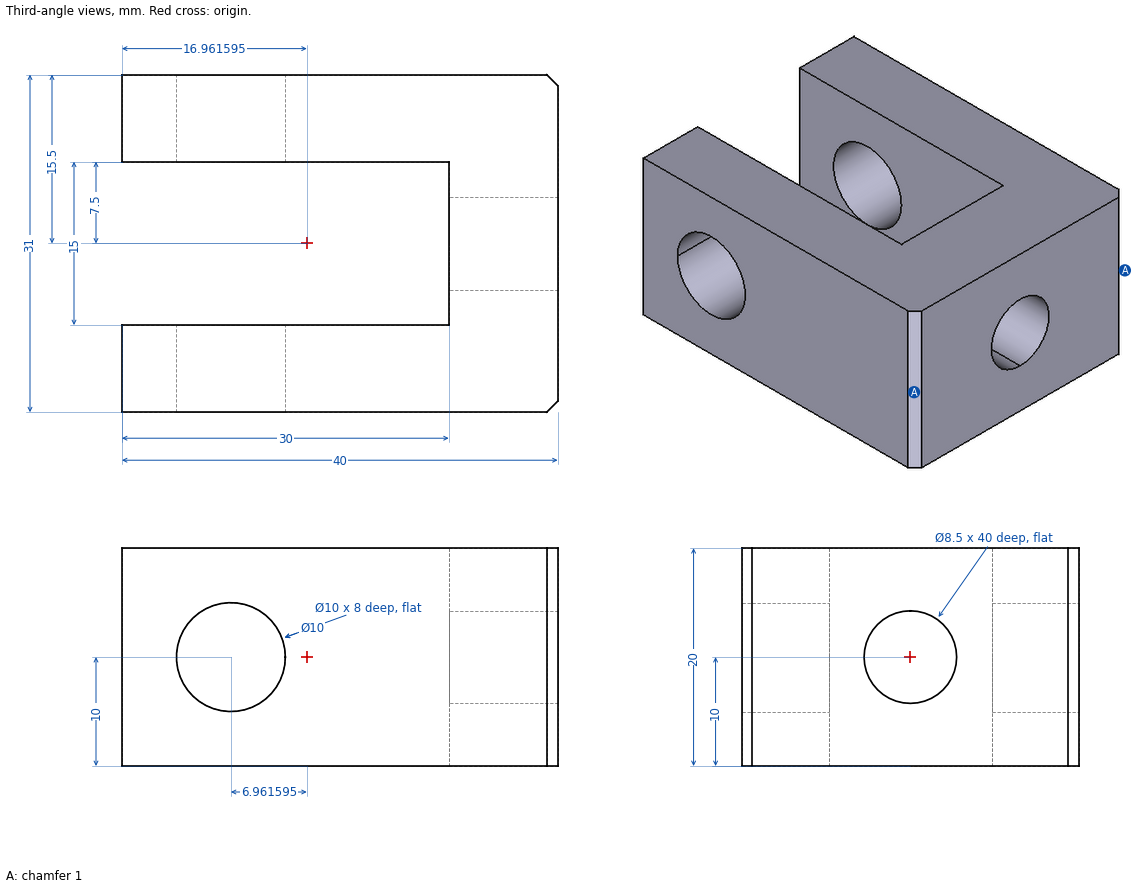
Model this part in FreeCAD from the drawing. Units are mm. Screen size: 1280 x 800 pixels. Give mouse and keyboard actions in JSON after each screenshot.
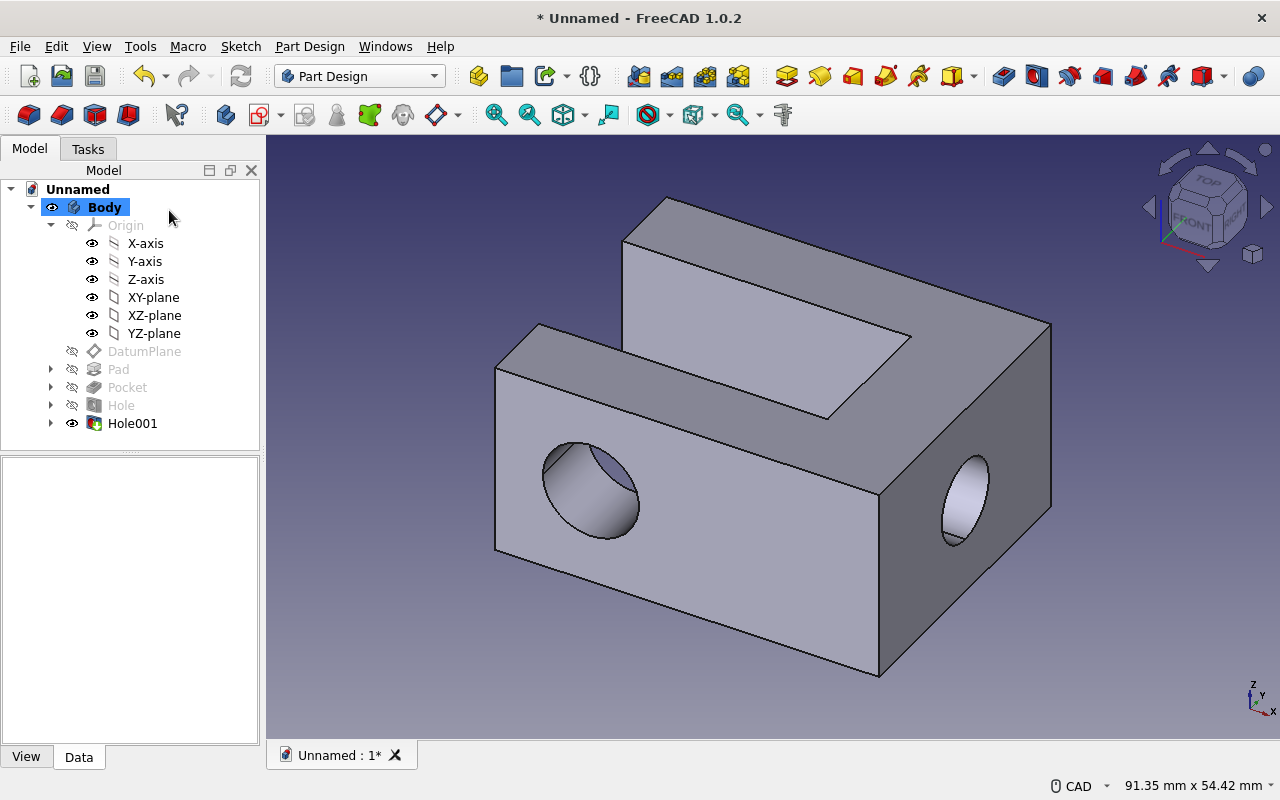
{"action": "left_click", "coordinate": [725, 365]}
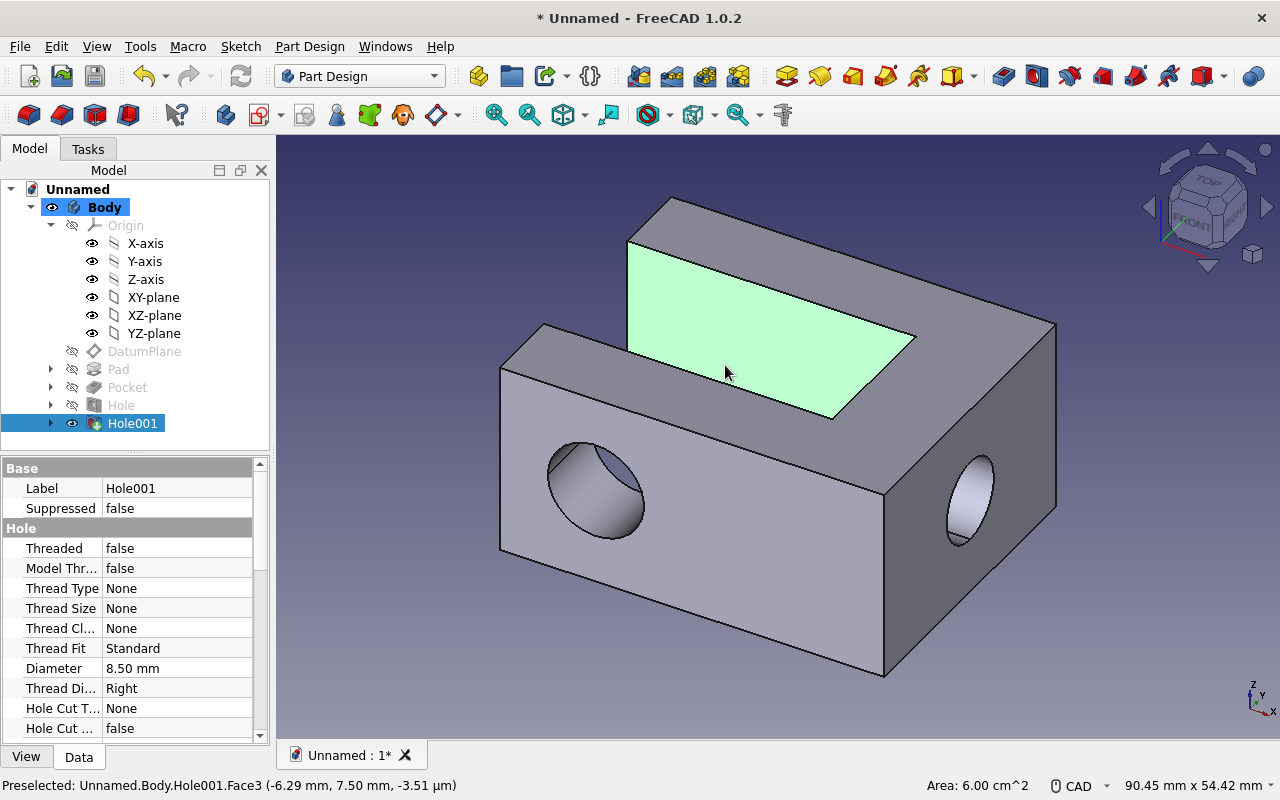
{"action": "left_click", "coordinate": [258, 116]}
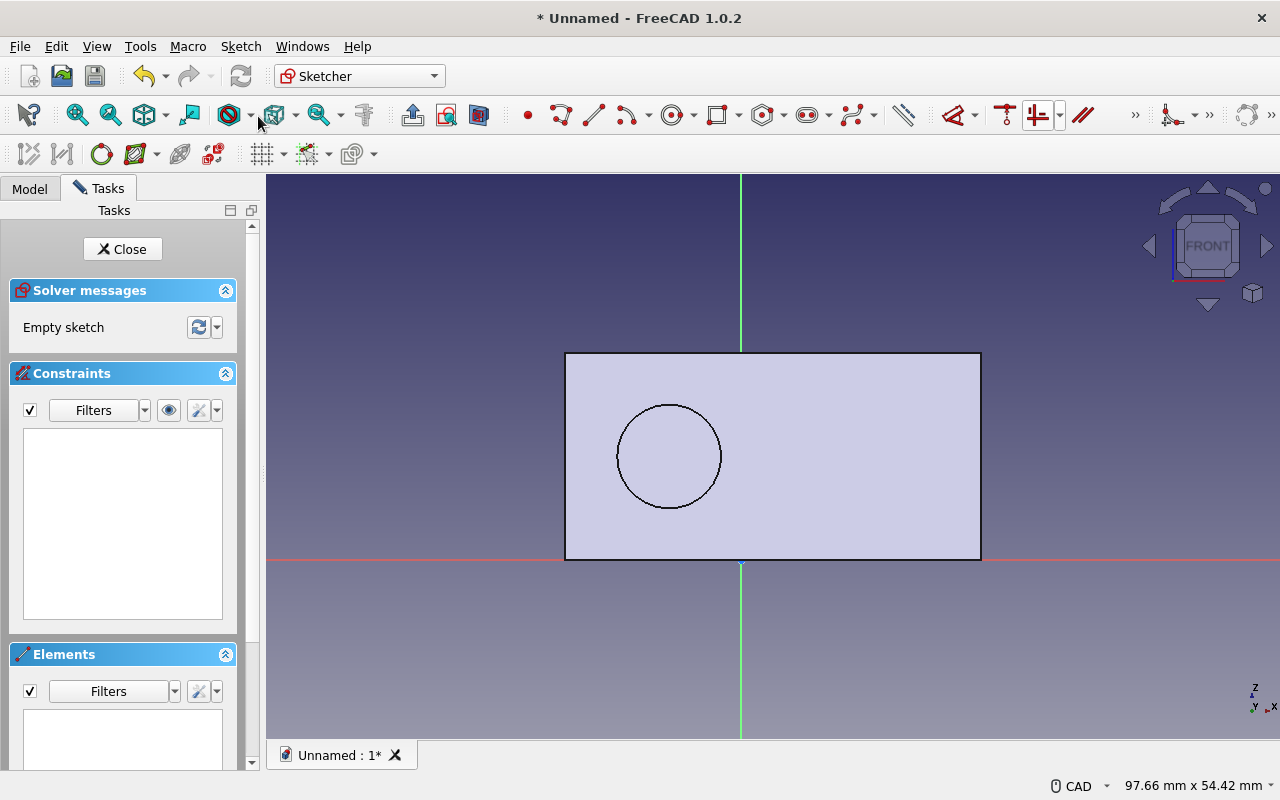
{"action": "scroll", "coordinate": [659, 504], "scroll_direction": "up", "scroll_amount": 4}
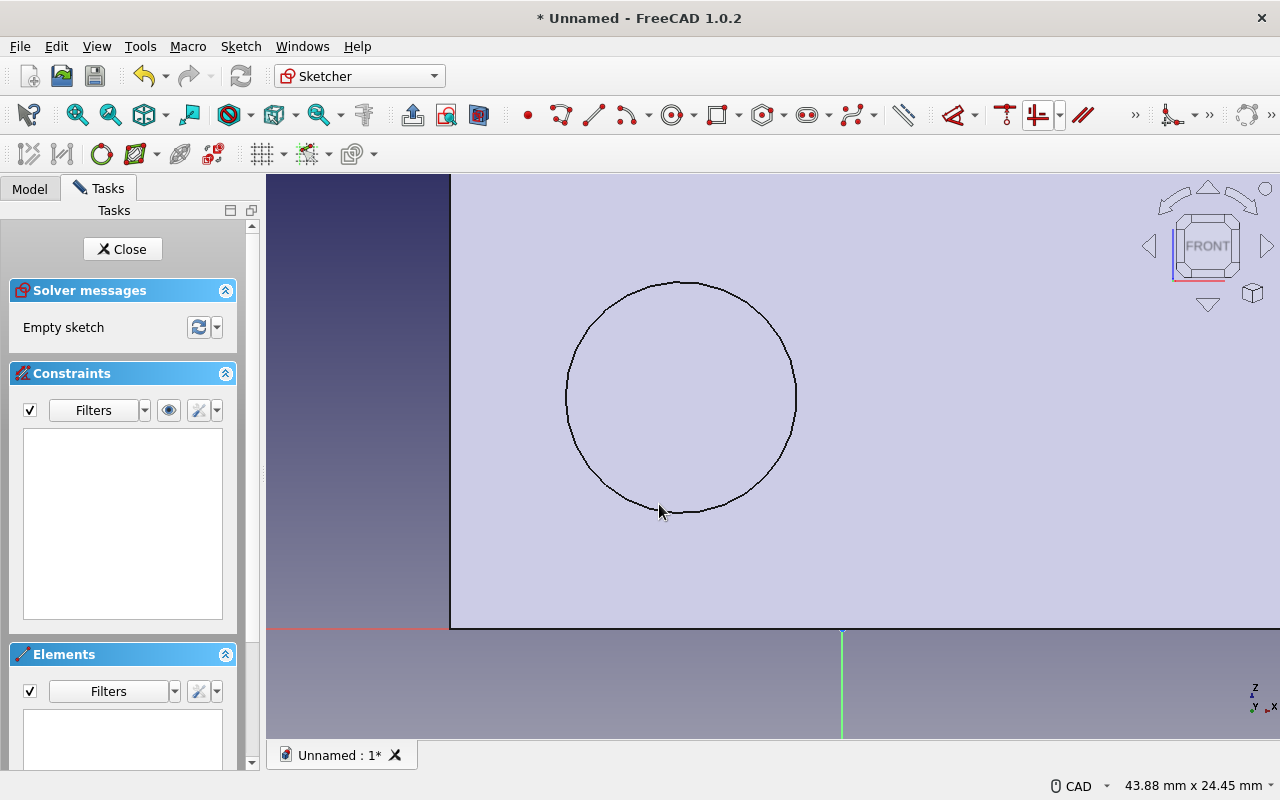
{"action": "key", "text": "g c"}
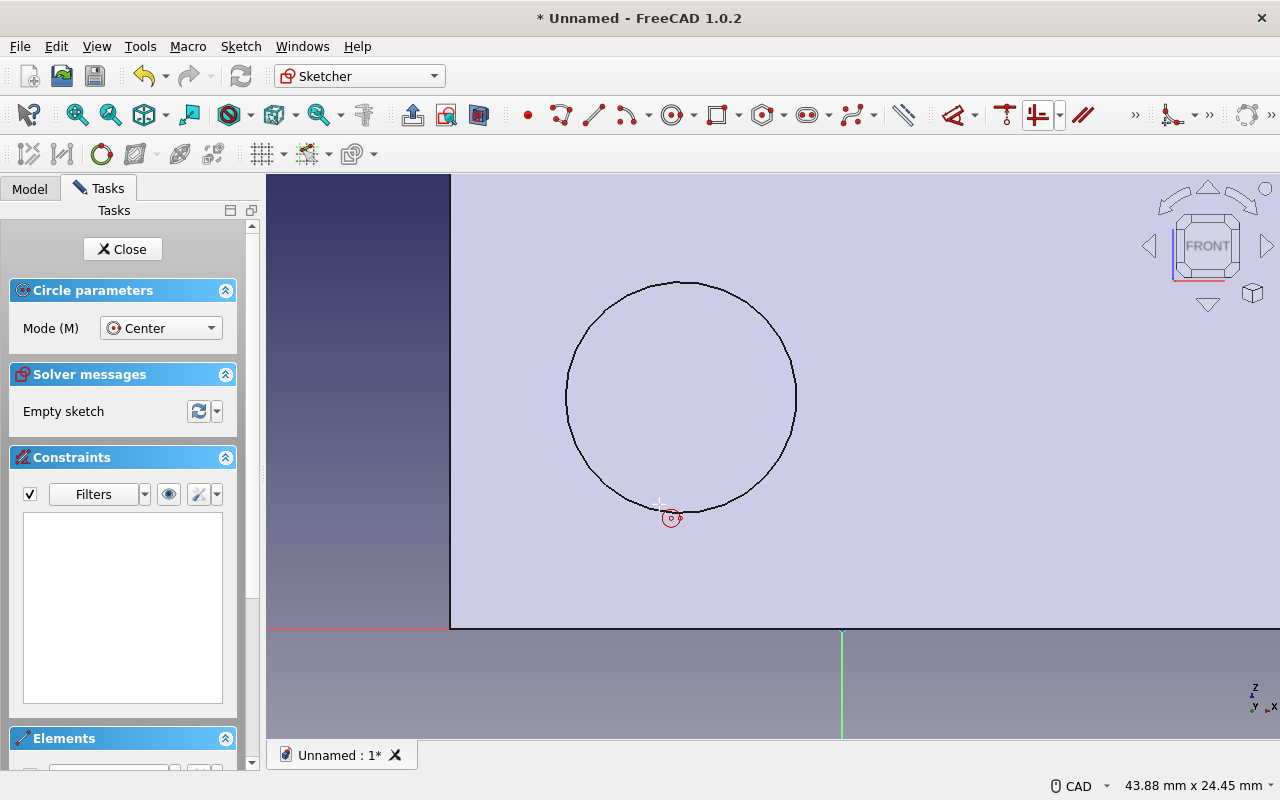
{"action": "left_click", "coordinate": [681, 398]}
{"action": "left_click", "coordinate": [763, 316]}
{"action": "key", "text": "Escape"}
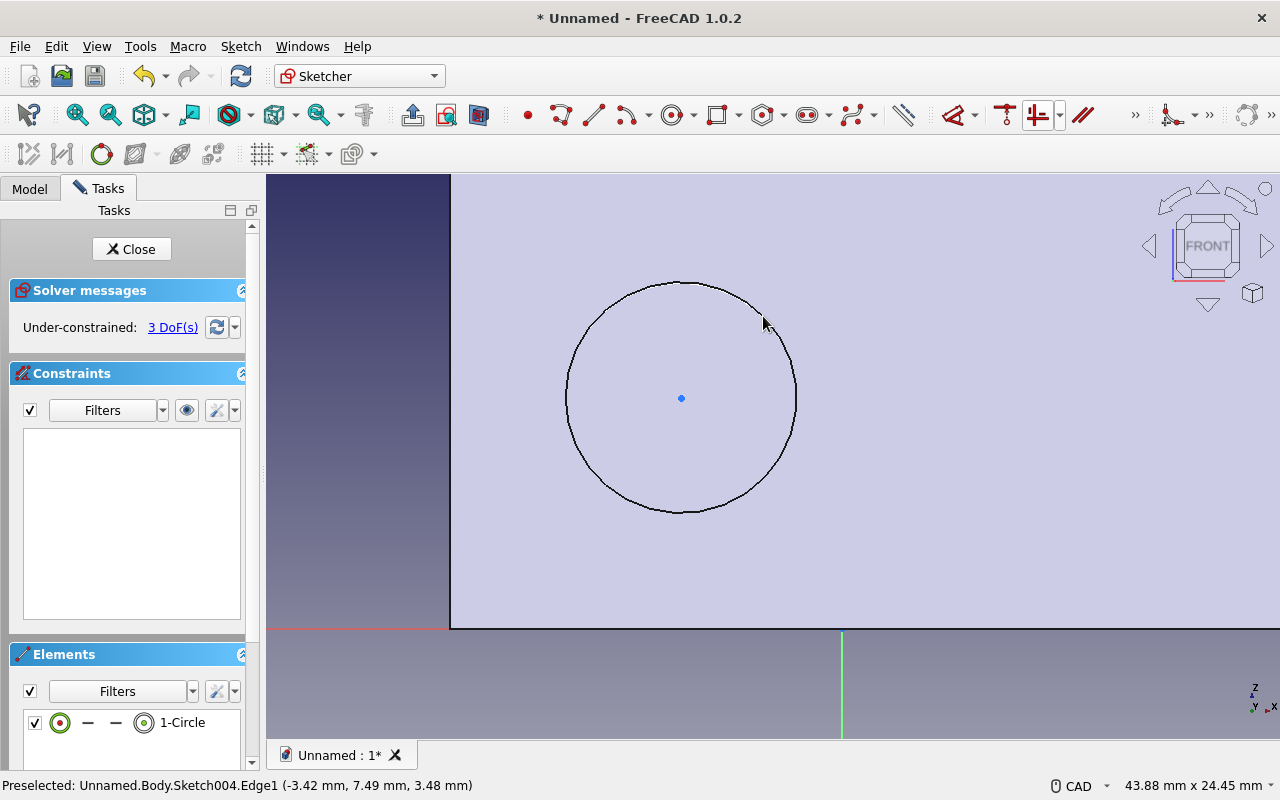
{"action": "left_click", "coordinate": [952, 116]}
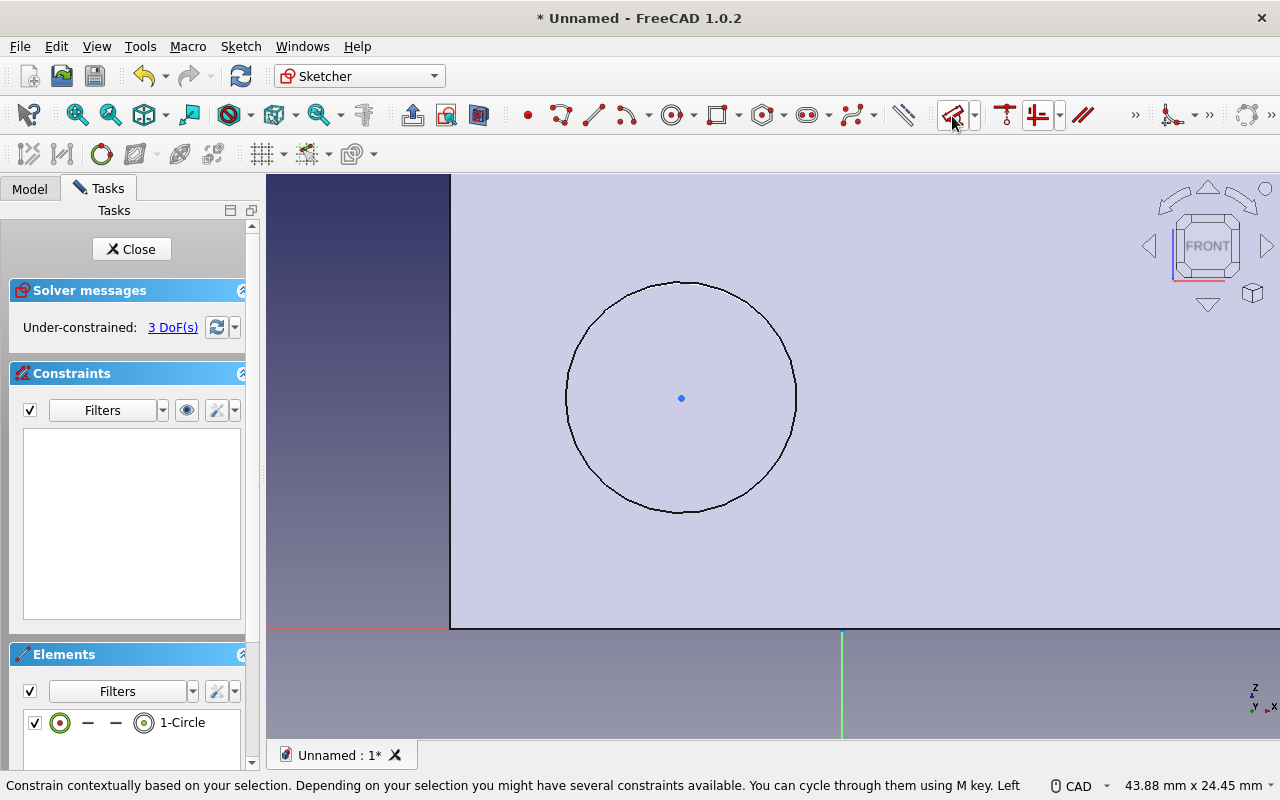
{"action": "left_click", "coordinate": [763, 317]}
{"action": "left_click", "coordinate": [786, 294]}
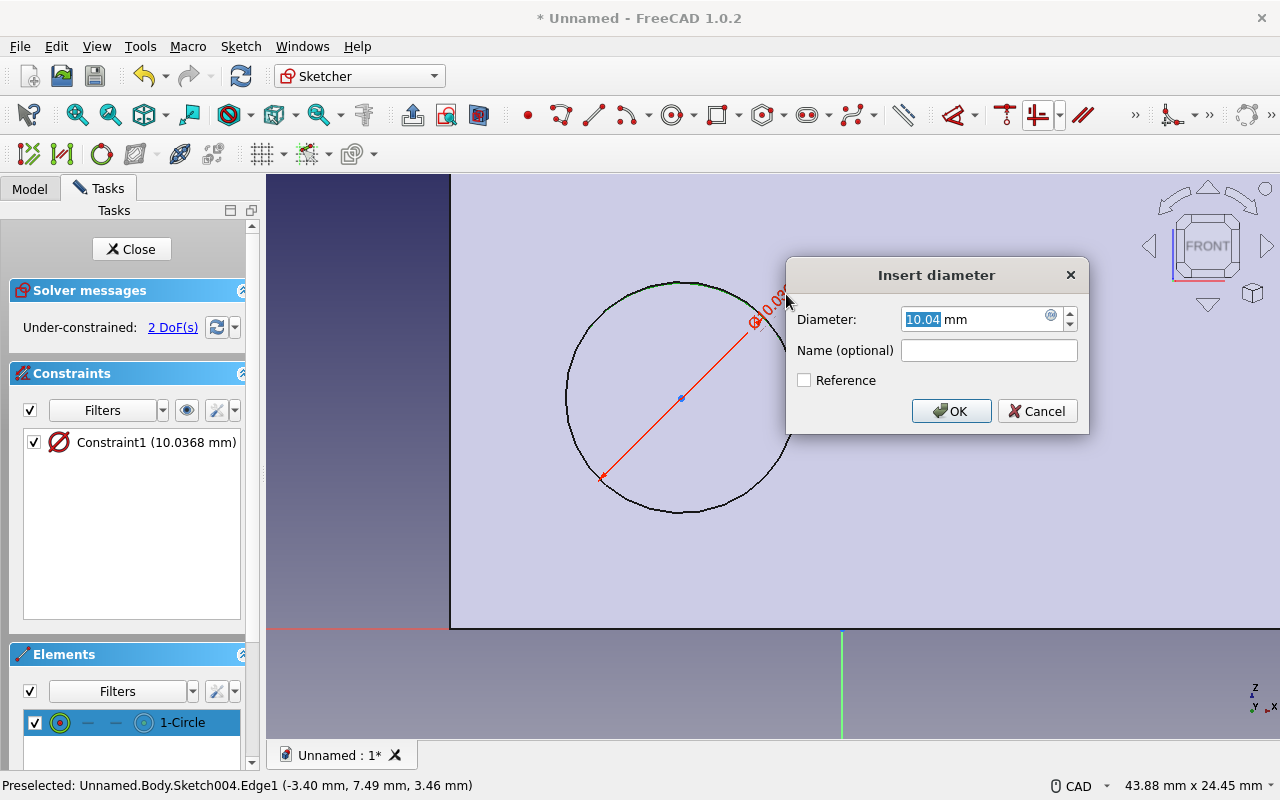
{"action": "type", "text": "10"}
{"action": "key", "text": "Return"}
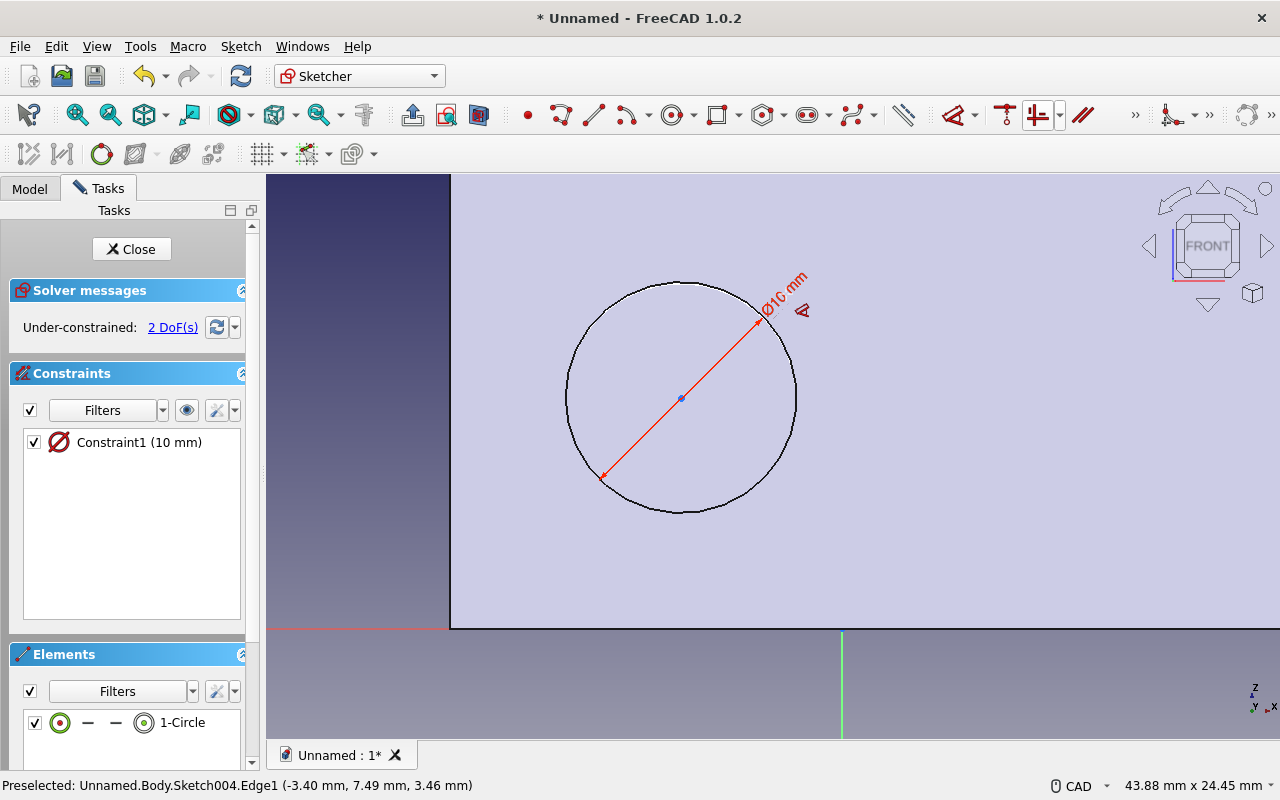
{"action": "left_click", "coordinate": [681, 399]}
{"action": "left_click", "coordinate": [876, 514]}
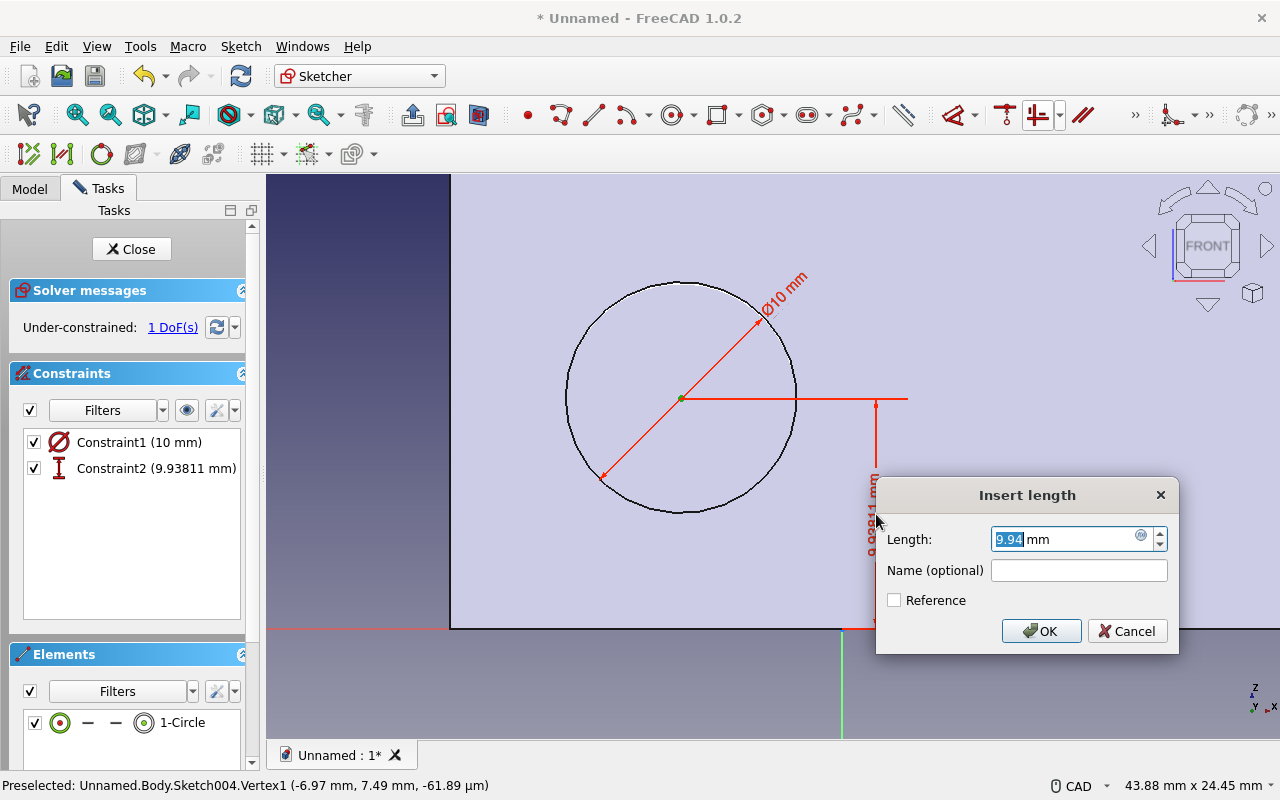
{"action": "type", "text": "10"}
{"action": "key", "text": "Return"}